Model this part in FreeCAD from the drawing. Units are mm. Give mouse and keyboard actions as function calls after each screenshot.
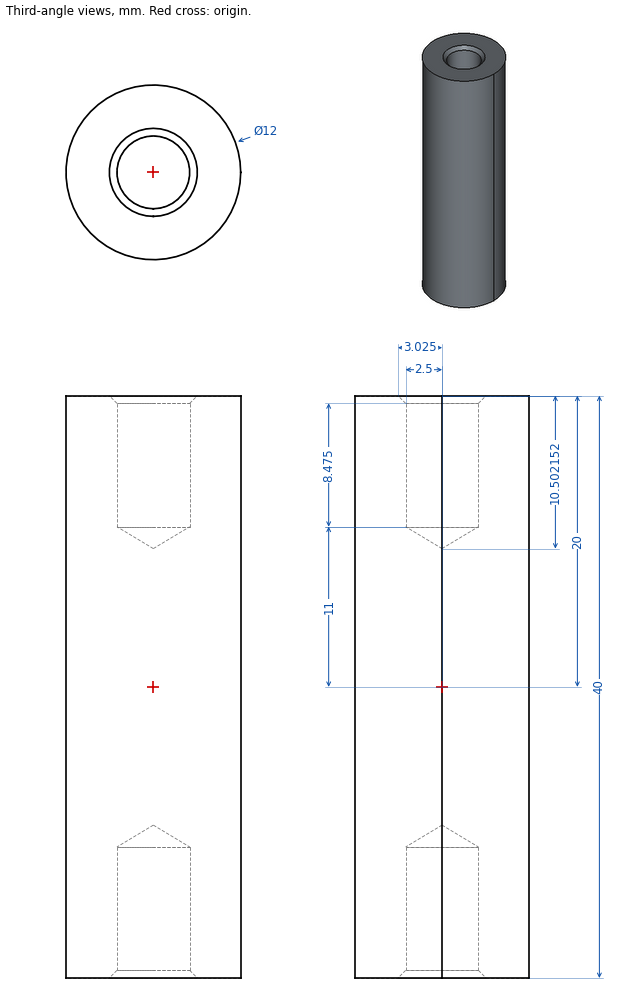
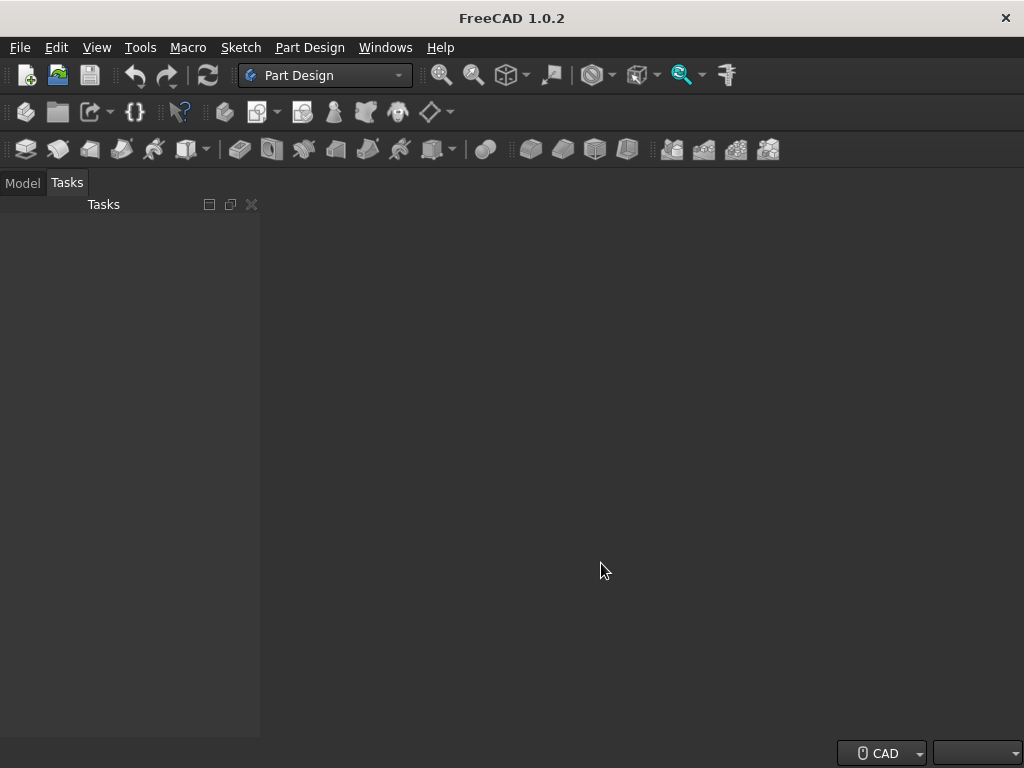
click(26, 76)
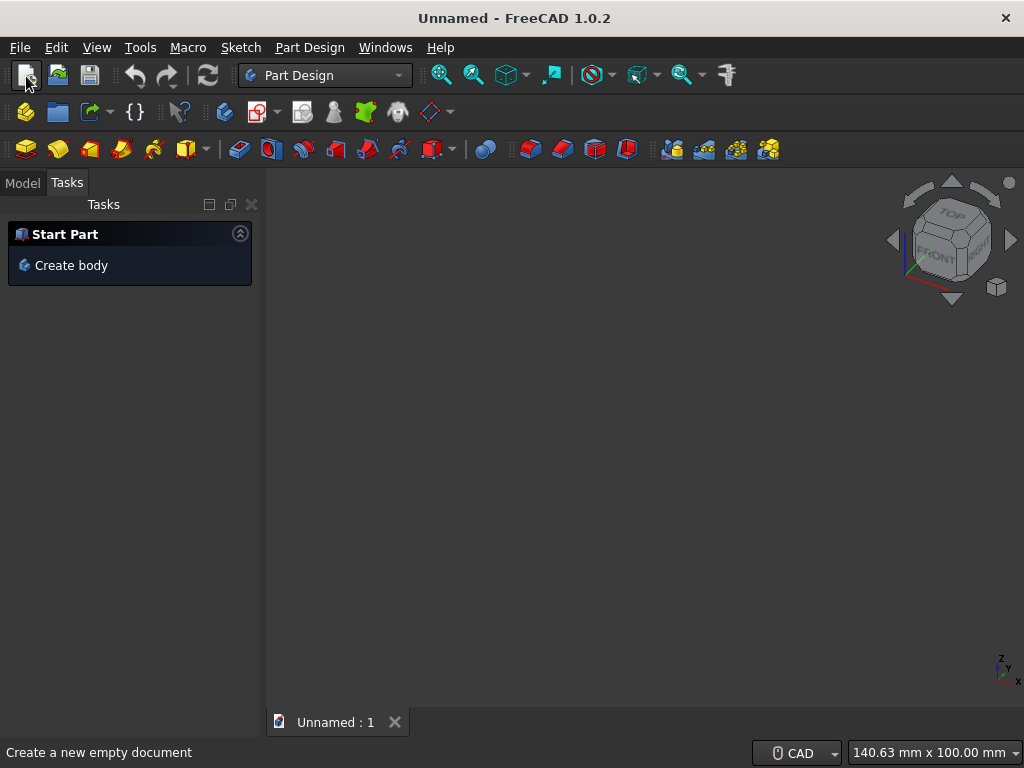
click(258, 112)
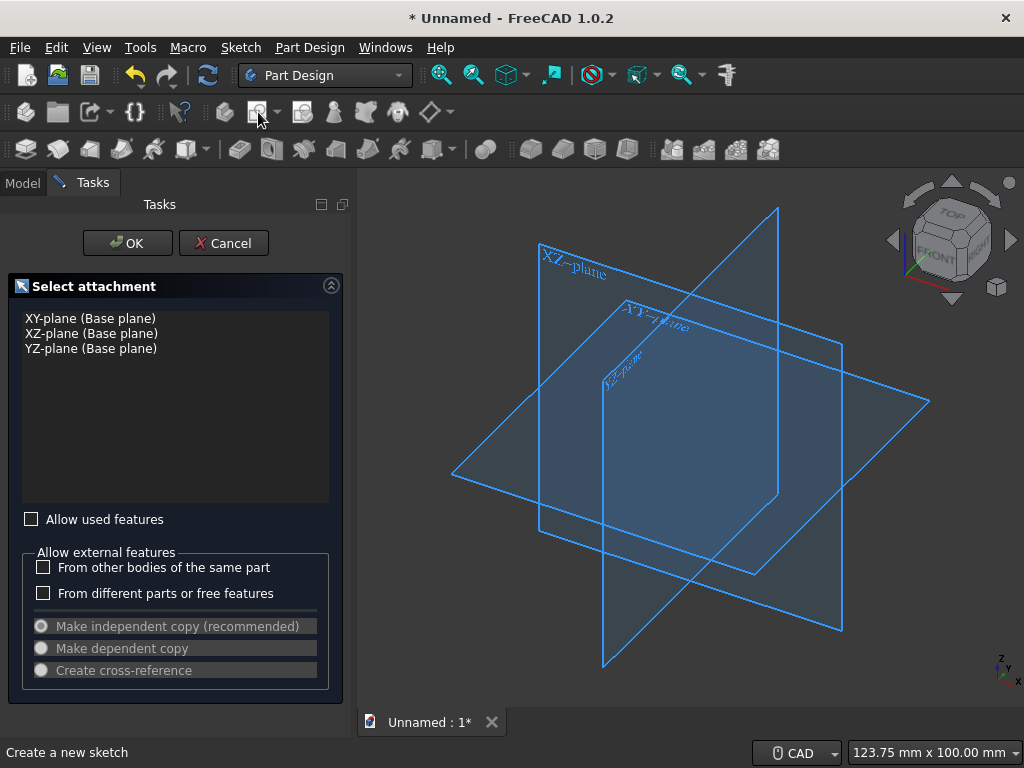
click(82, 318)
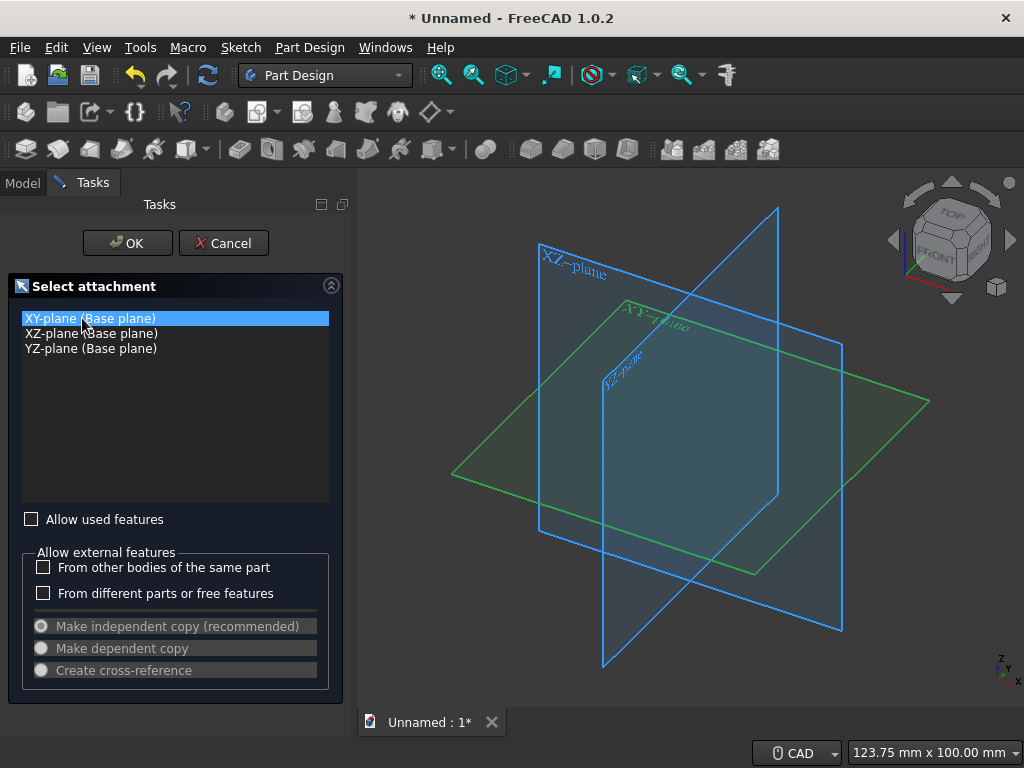
click(128, 243)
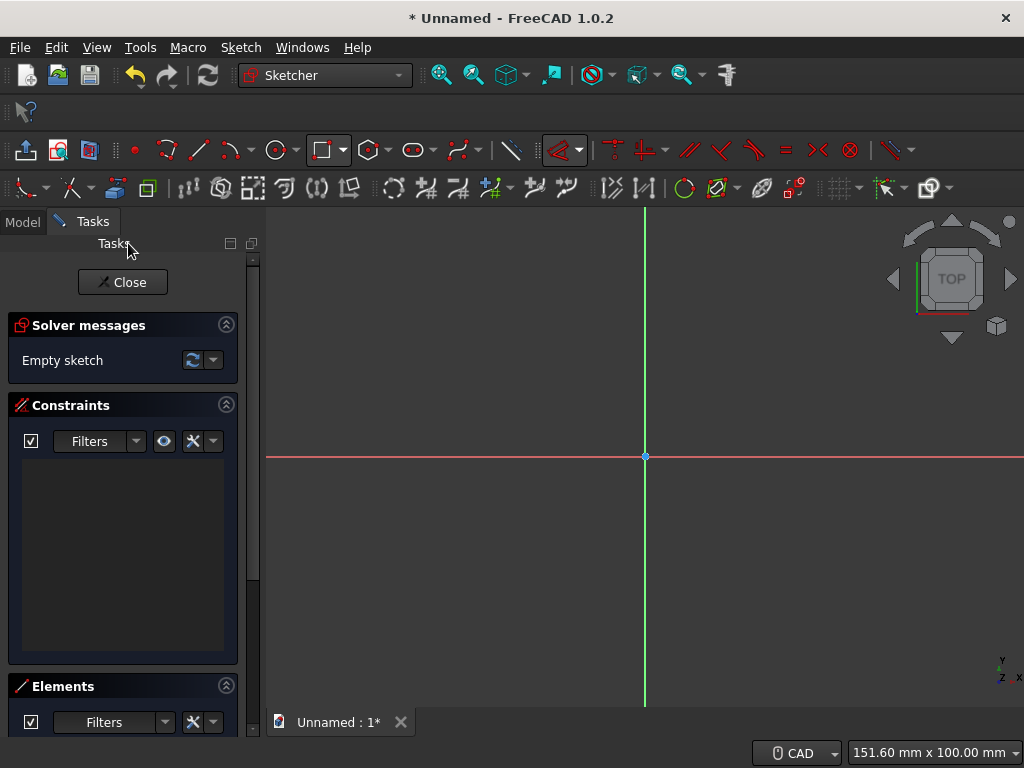
scroll(662, 457, up, 8)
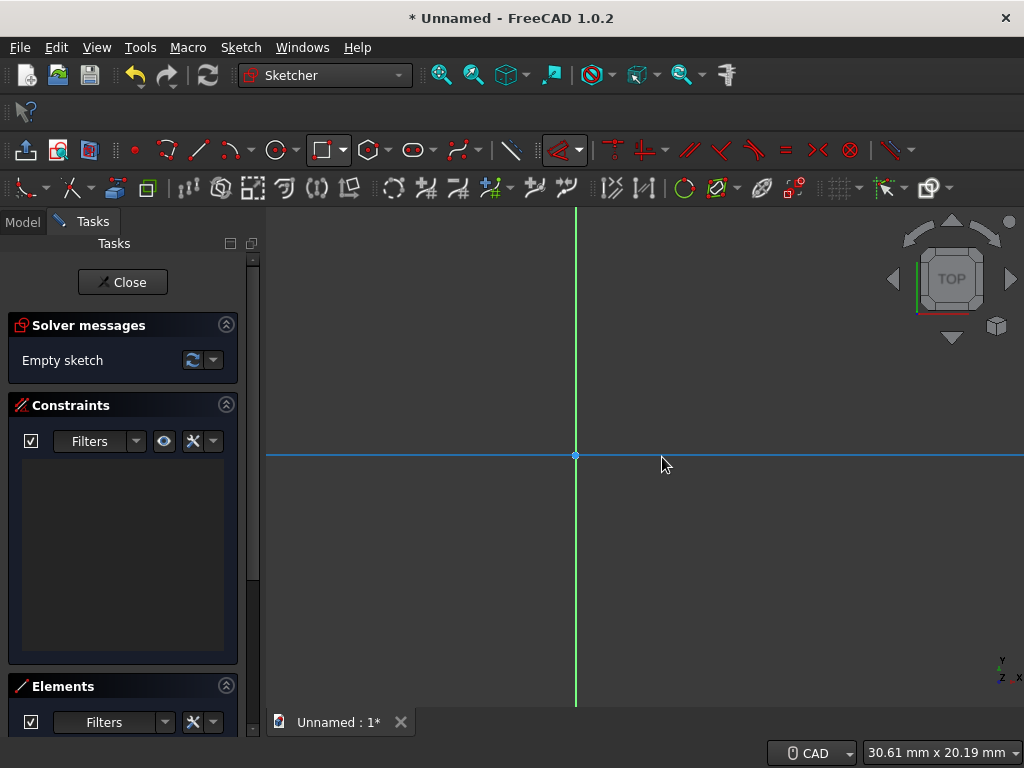
click(276, 150)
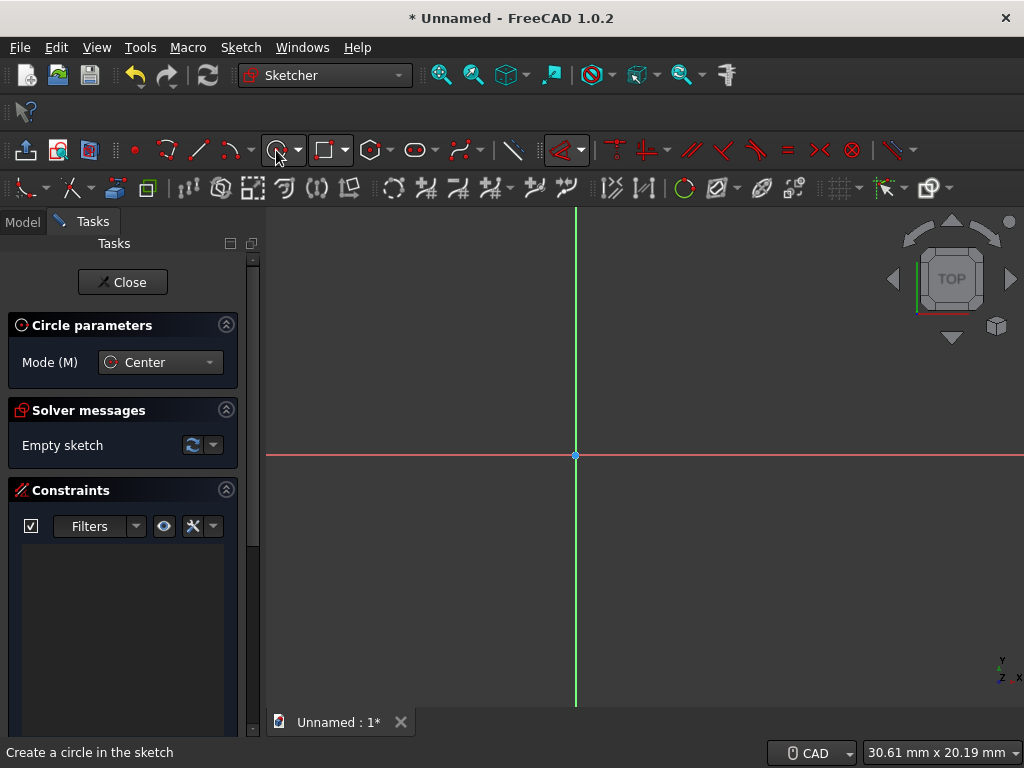
click(576, 455)
click(681, 350)
key(Escape)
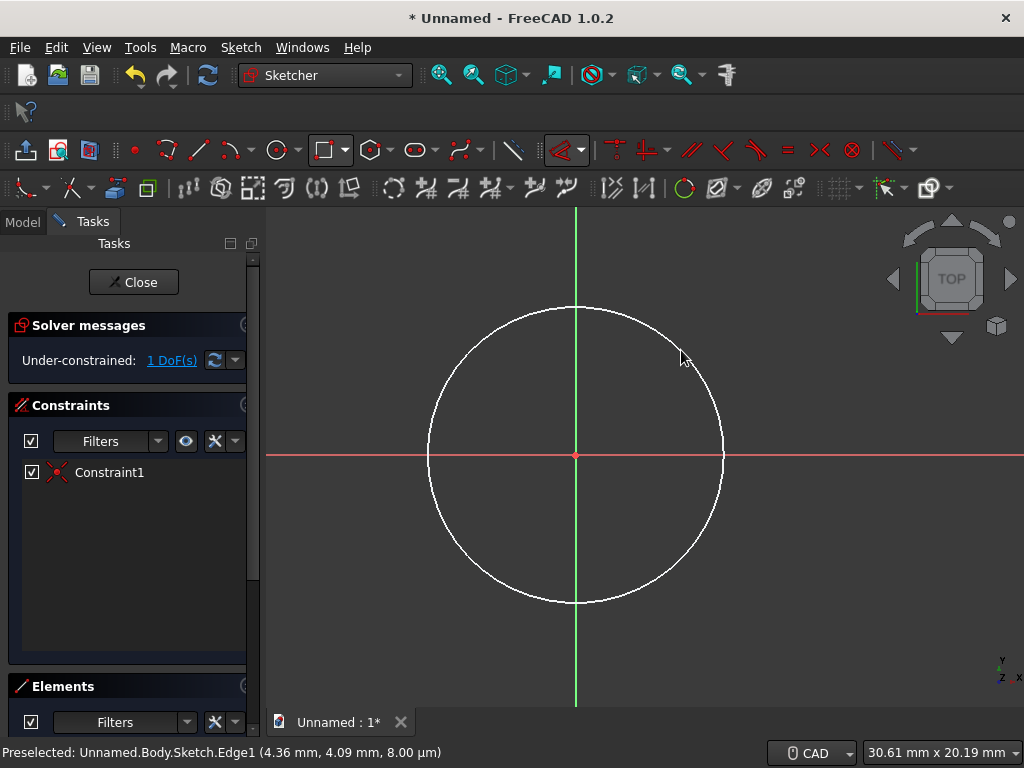
click(680, 350)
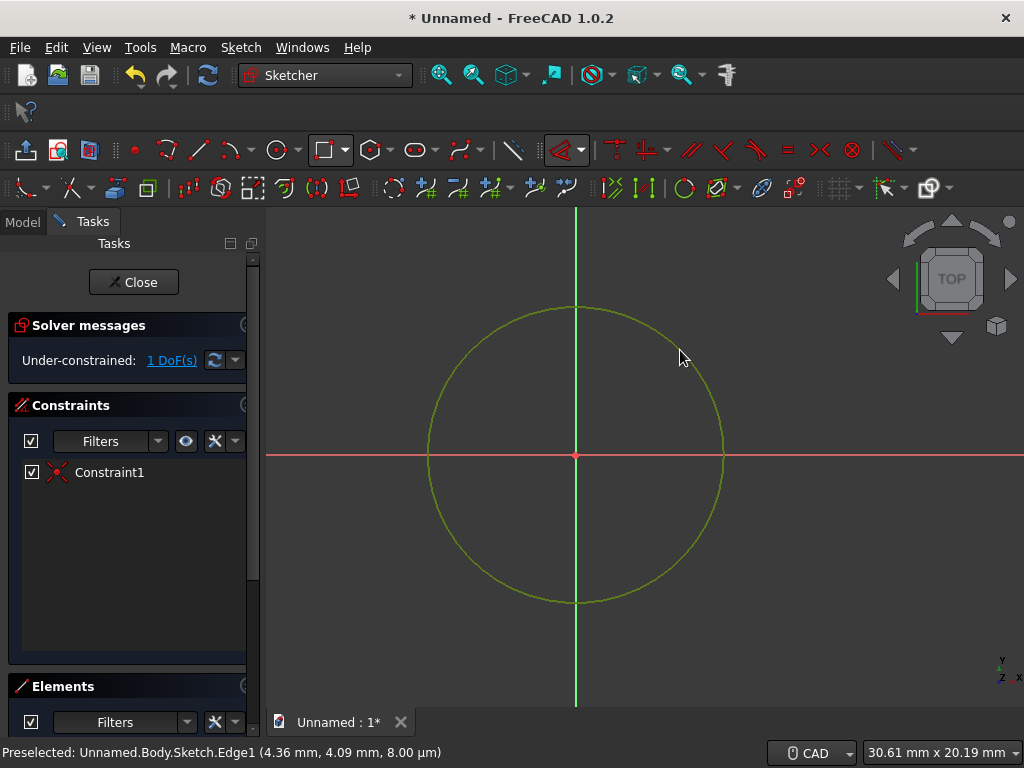
key(k)
key(o)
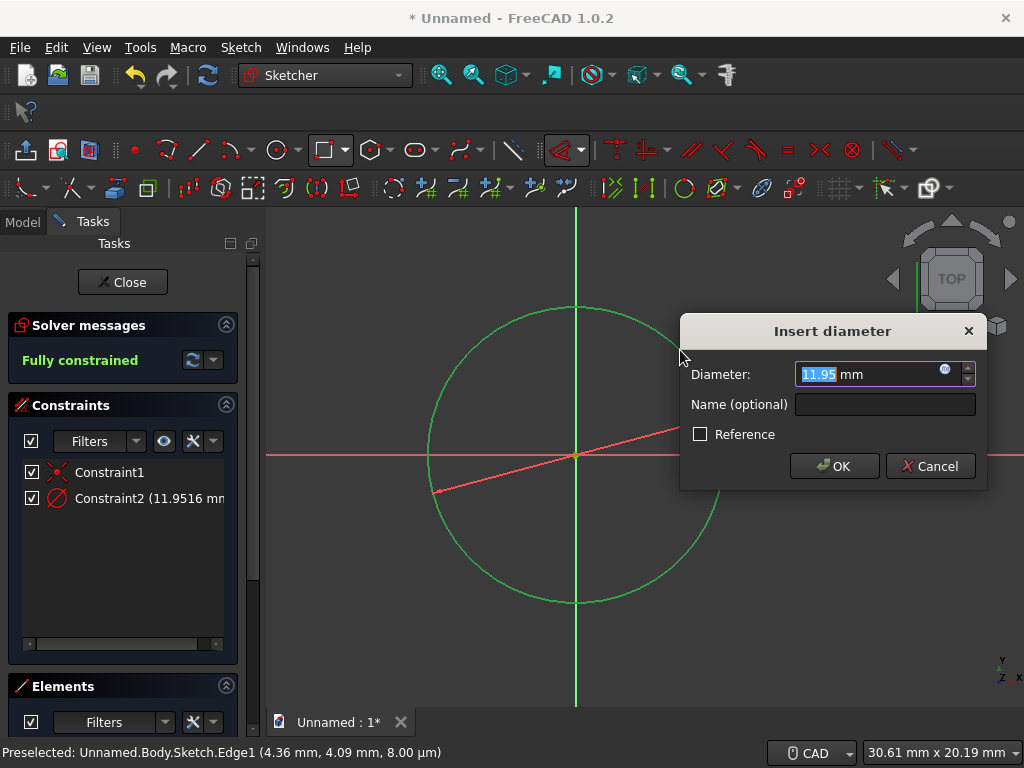
text(12)
key(Return)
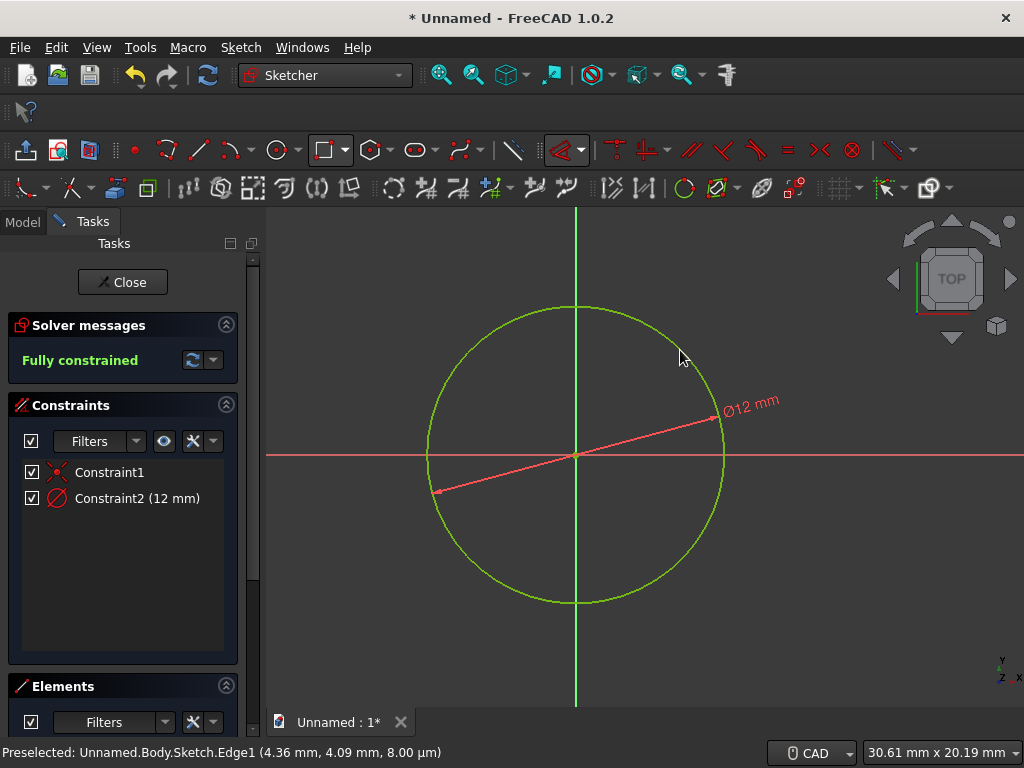
click(123, 282)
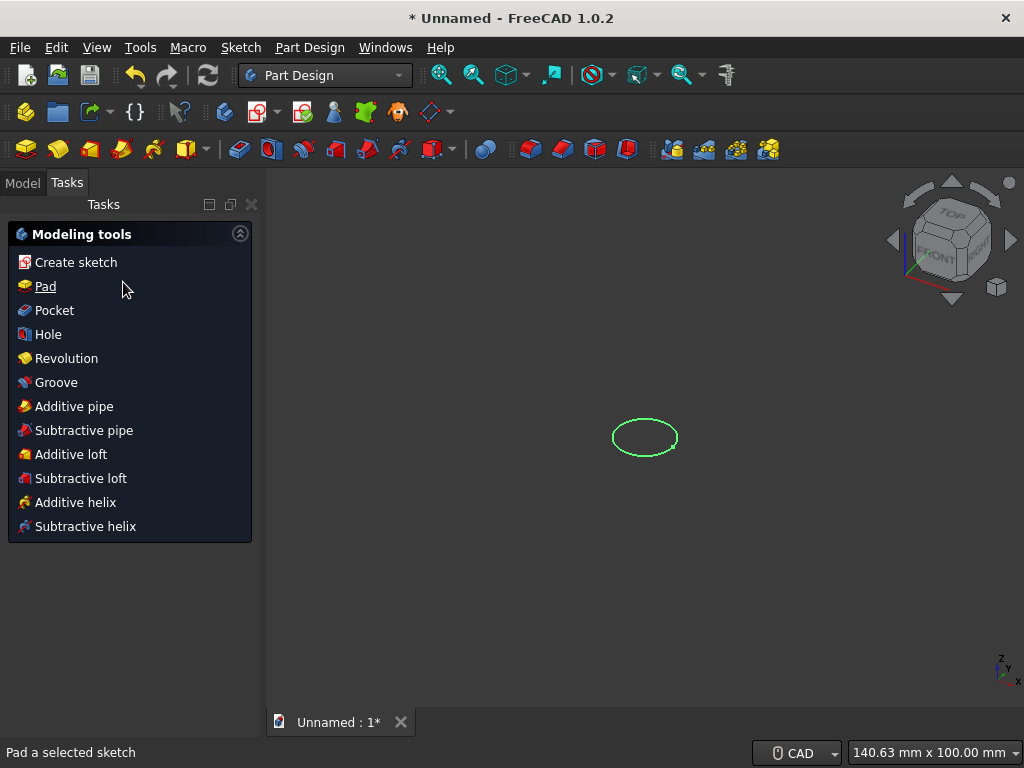
click(26, 150)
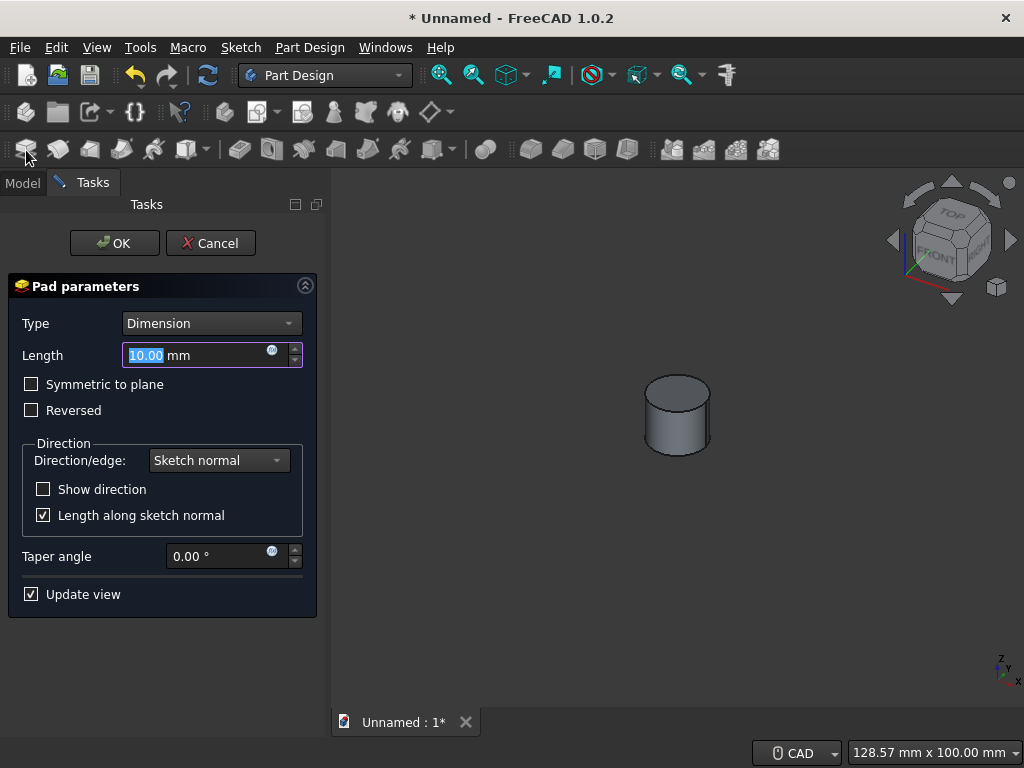
text(40)
key(Tab)